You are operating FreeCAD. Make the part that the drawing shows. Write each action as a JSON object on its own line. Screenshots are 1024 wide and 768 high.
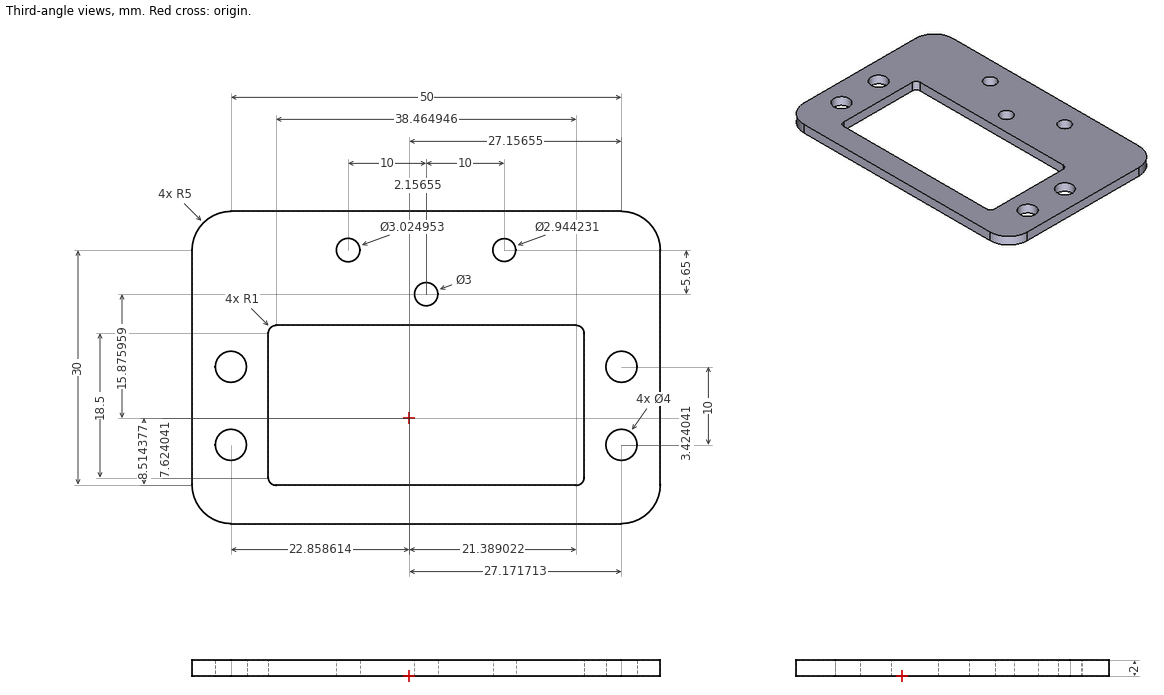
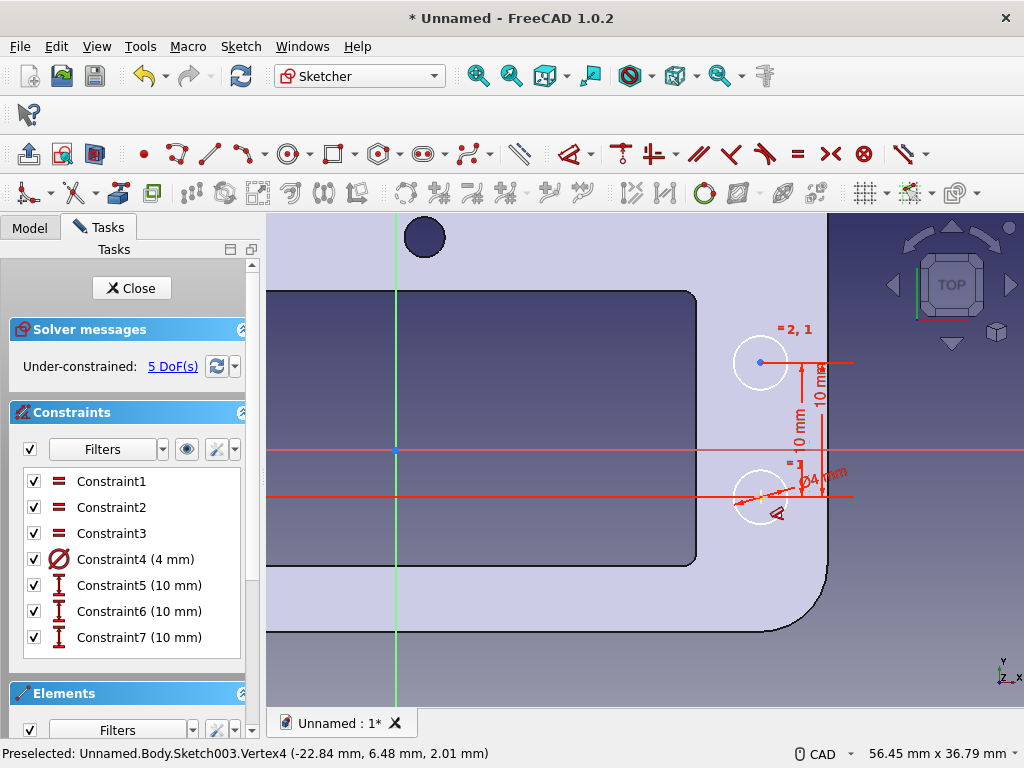
{"action": "left_click", "coordinate": [761, 497]}
{"action": "left_click", "coordinate": [362, 474]}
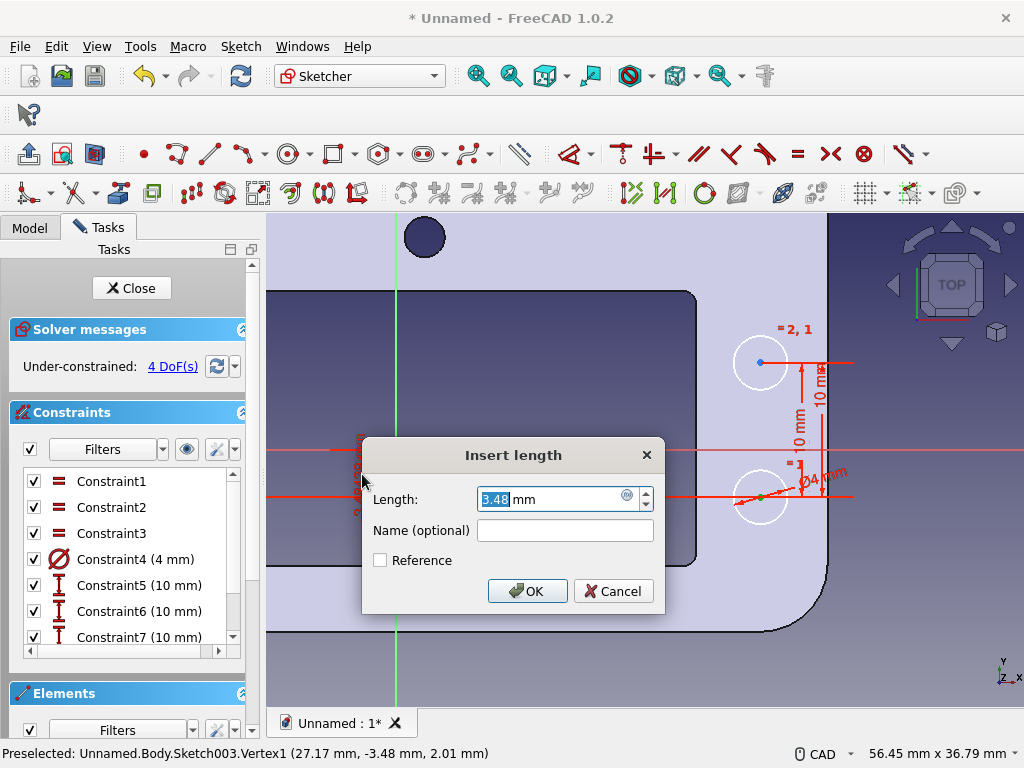
{"action": "type", "text": "3.424041"}
{"action": "key", "text": "Return"}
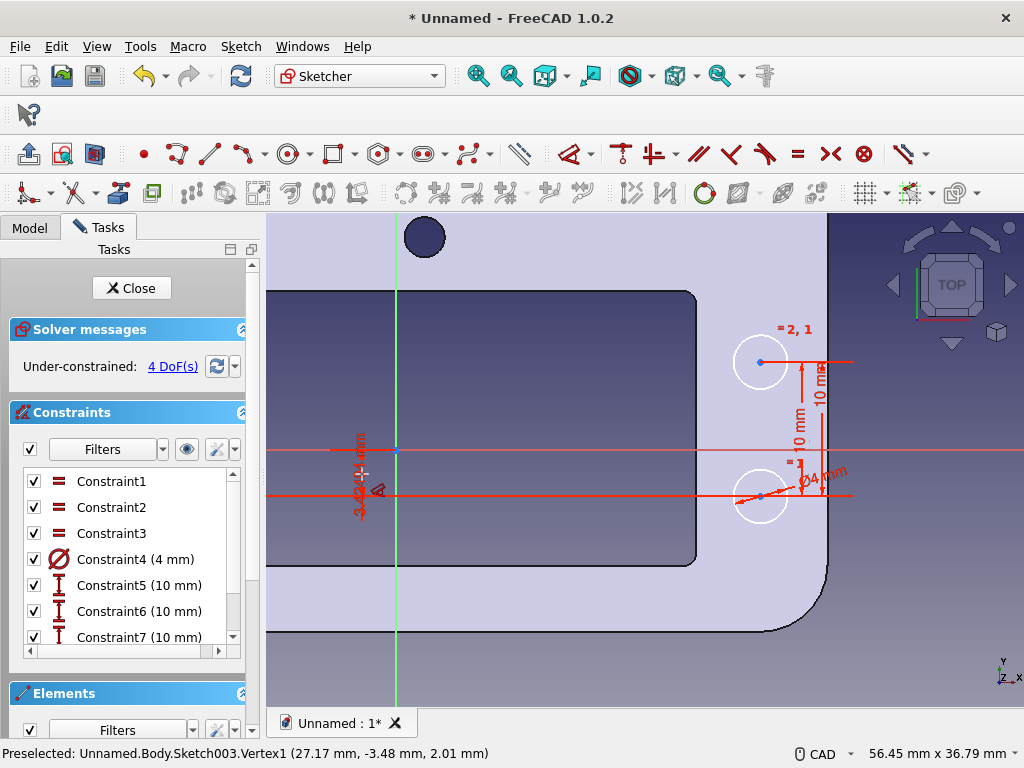
{"action": "left_click", "coordinate": [761, 496]}
{"action": "left_click", "coordinate": [578, 530]}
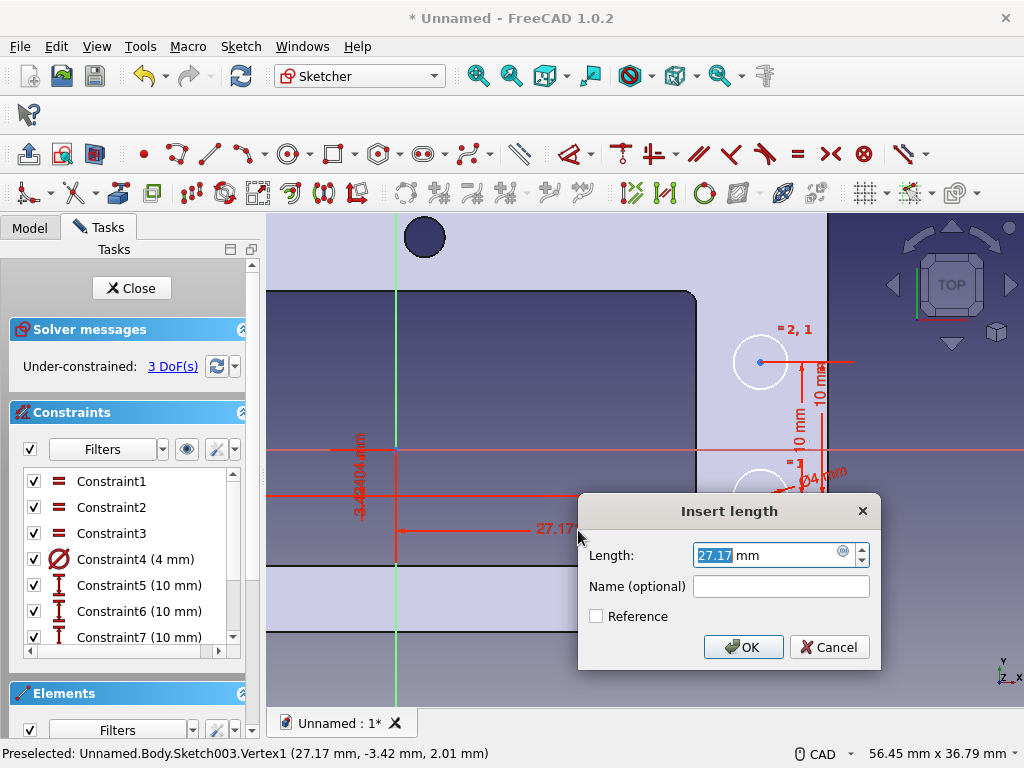
{"action": "type", "text": "27.171713"}
{"action": "key", "text": "Return"}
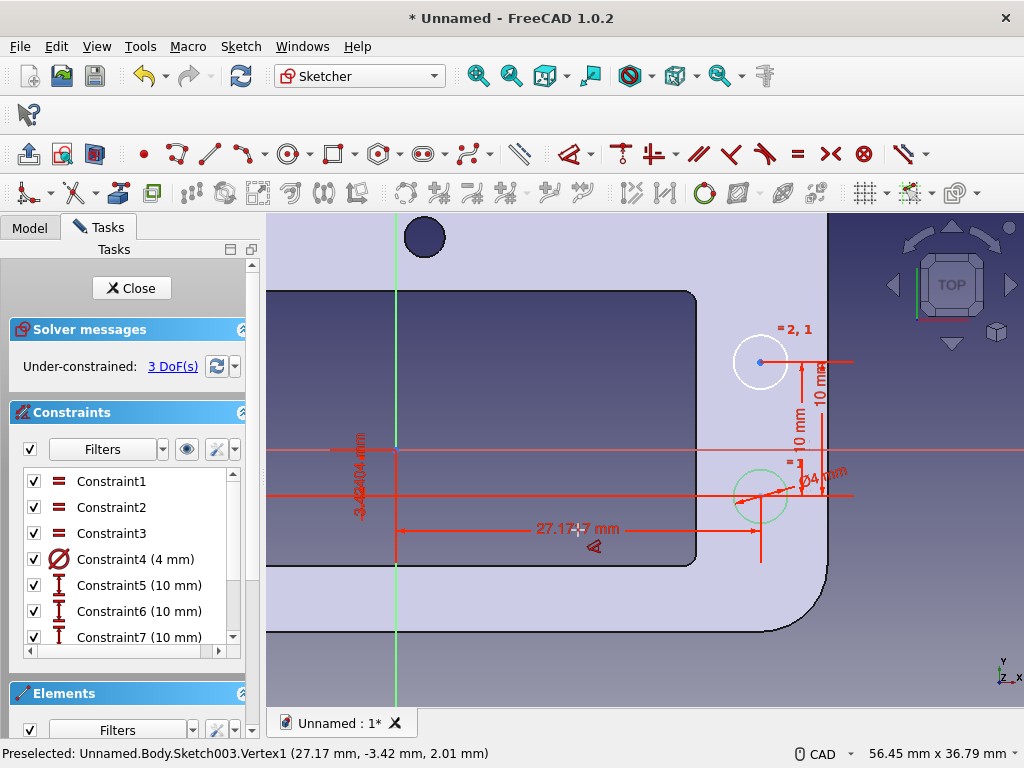
{"action": "left_click", "coordinate": [761, 362]}
{"action": "left_click", "coordinate": [578, 328]}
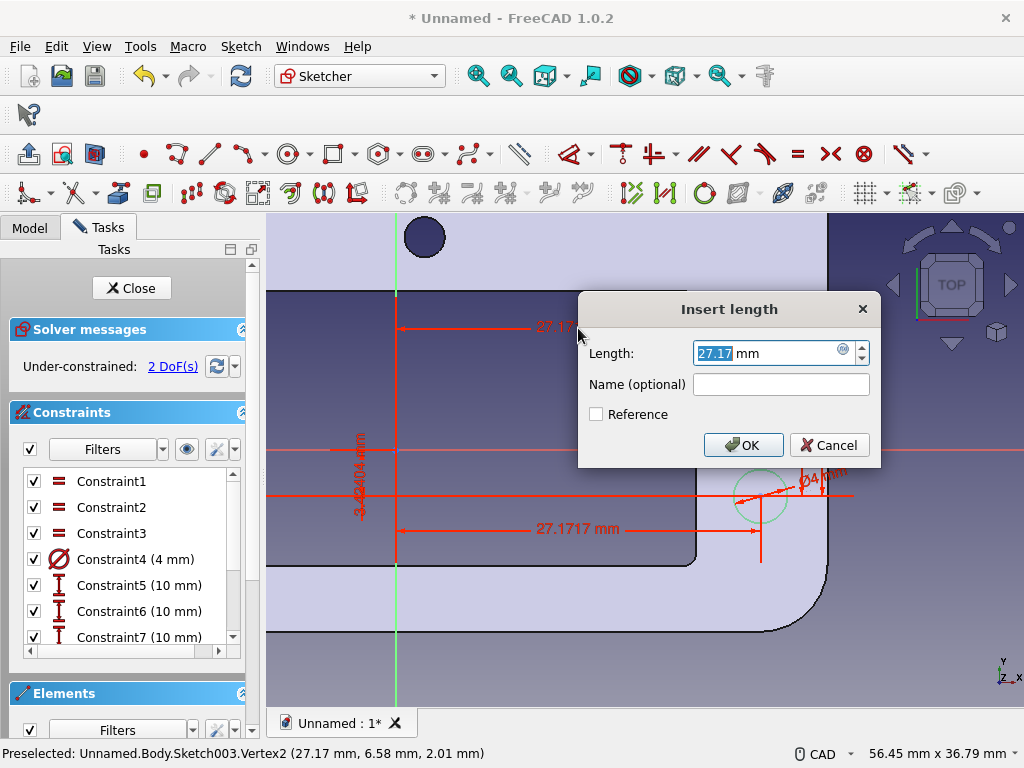
{"action": "type", "text": "27.171713"}
{"action": "key", "text": "Return"}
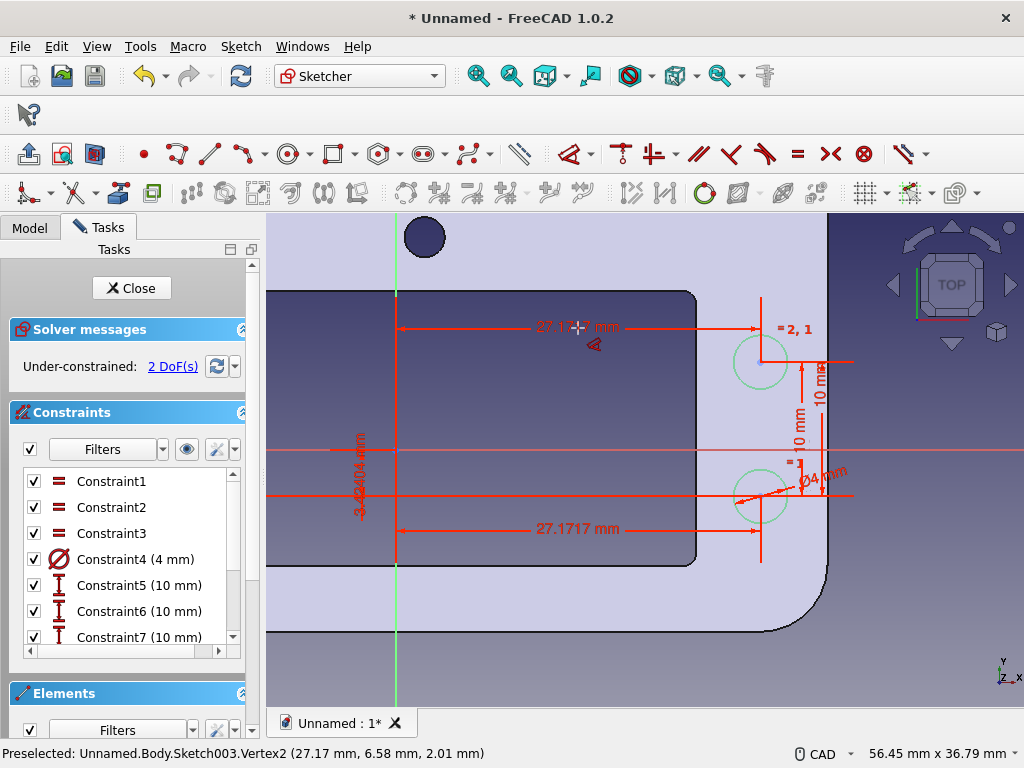
{"action": "scroll", "coordinate": [761, 497], "scroll_direction": "down", "scroll_amount": 3}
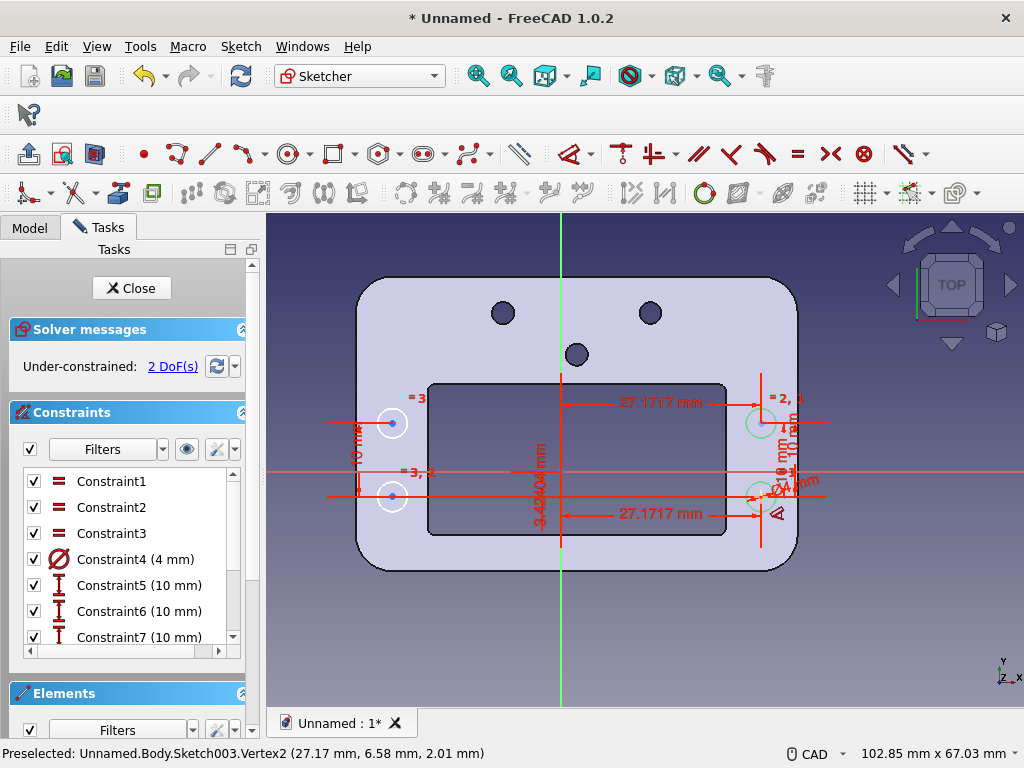
{"action": "left_click", "coordinate": [393, 497]}
{"action": "left_click", "coordinate": [477, 531]}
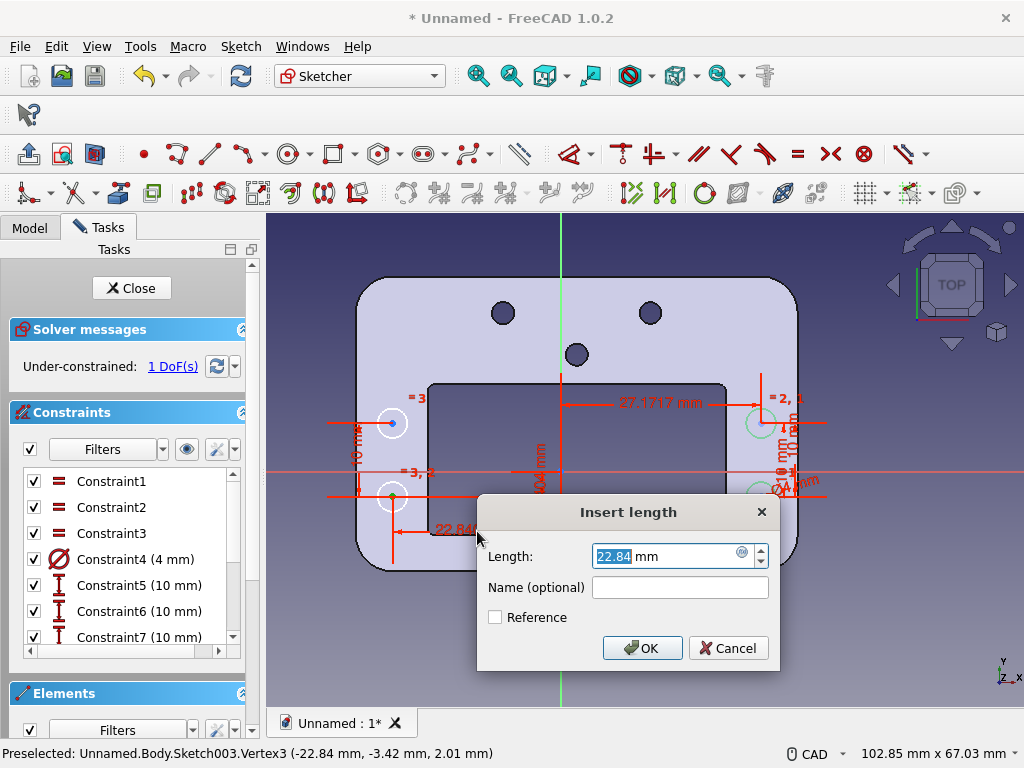
{"action": "type", "text": "22.858614"}
{"action": "key", "text": "Return"}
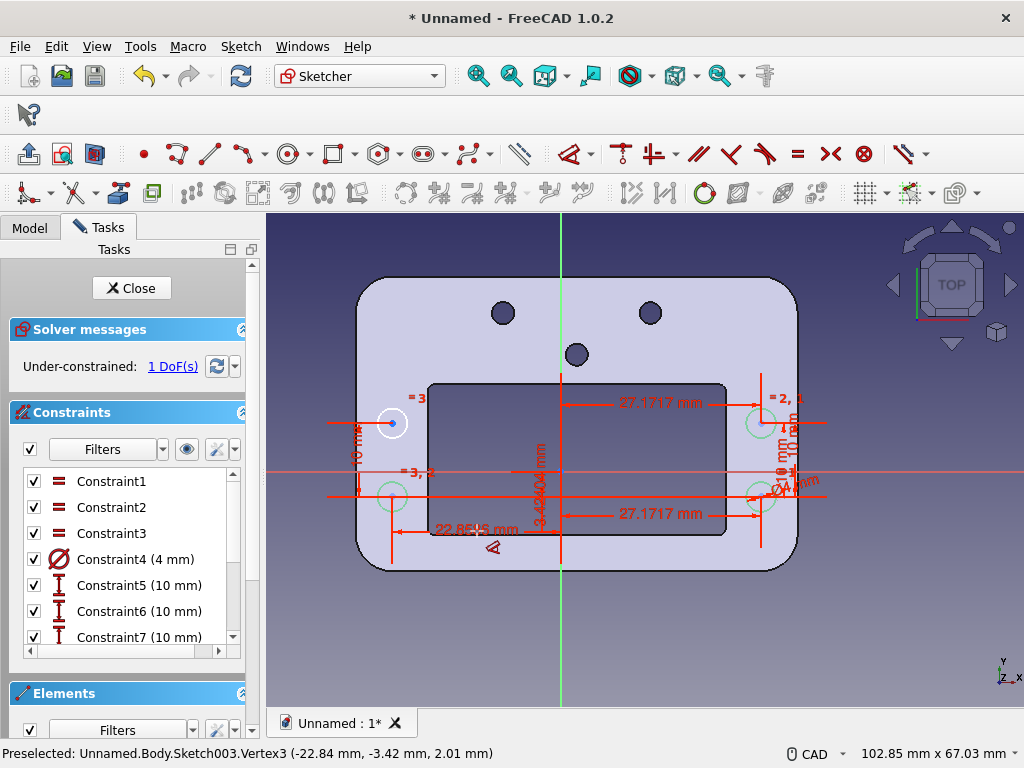
{"action": "left_click", "coordinate": [393, 423]}
{"action": "left_click", "coordinate": [477, 389]}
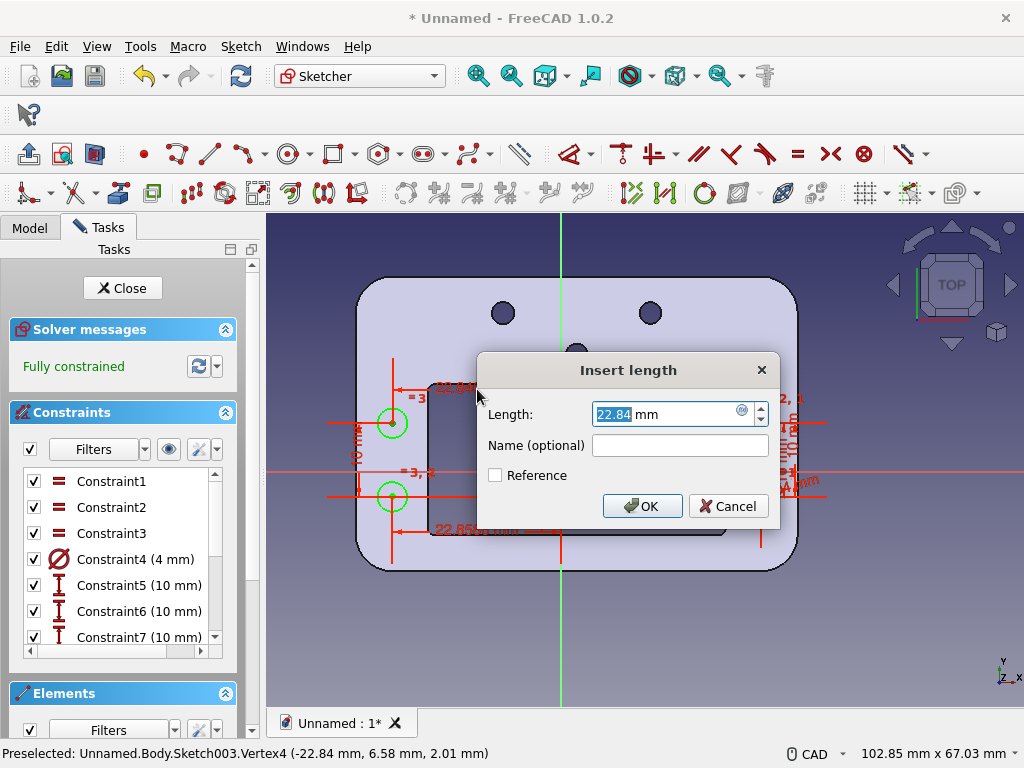
{"action": "type", "text": "22.858614"}
{"action": "key", "text": "Return"}
{"action": "key", "text": "Escape"}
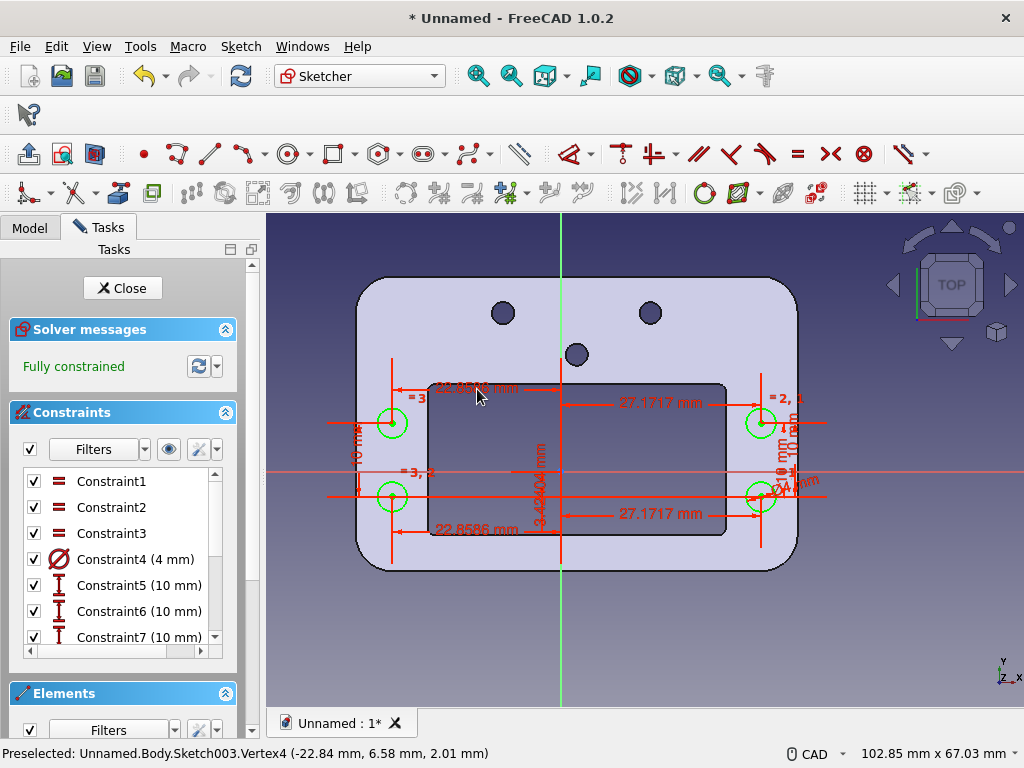
{"action": "left_click", "coordinate": [123, 288]}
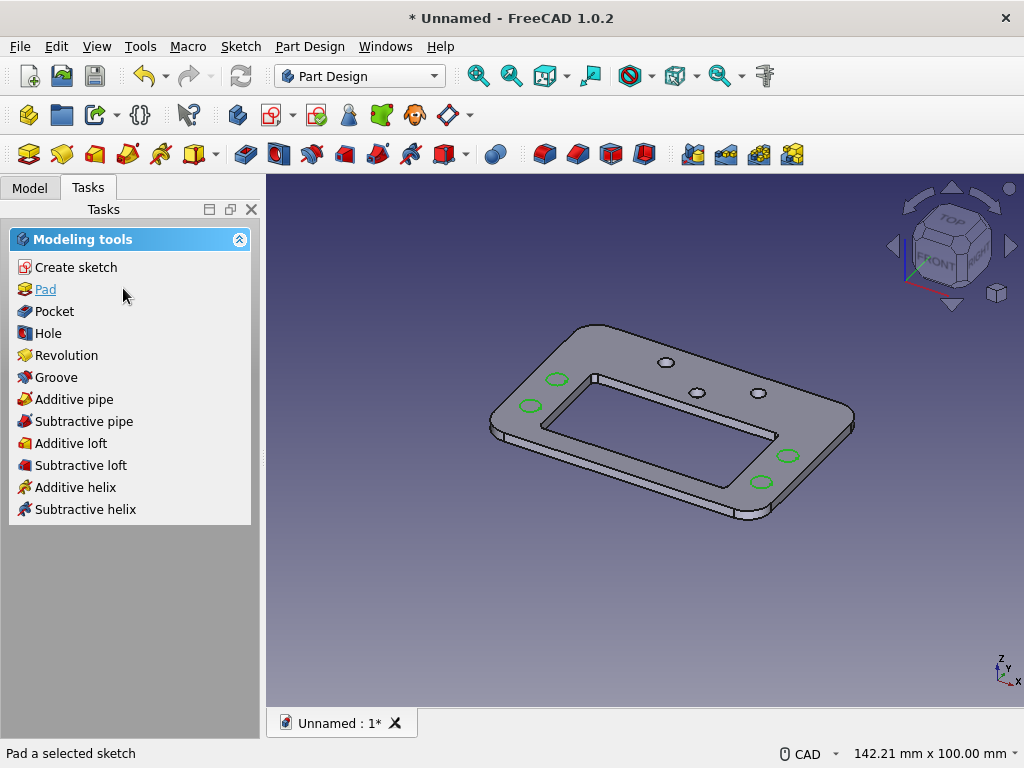
{"action": "left_click", "coordinate": [246, 154]}